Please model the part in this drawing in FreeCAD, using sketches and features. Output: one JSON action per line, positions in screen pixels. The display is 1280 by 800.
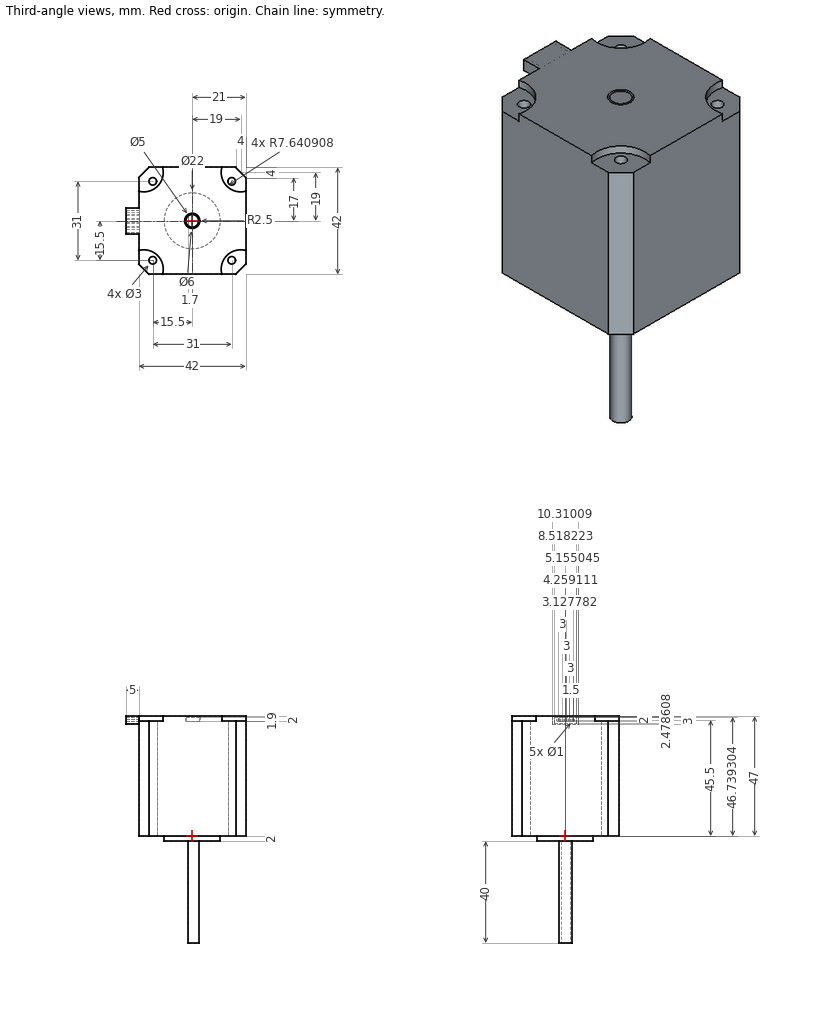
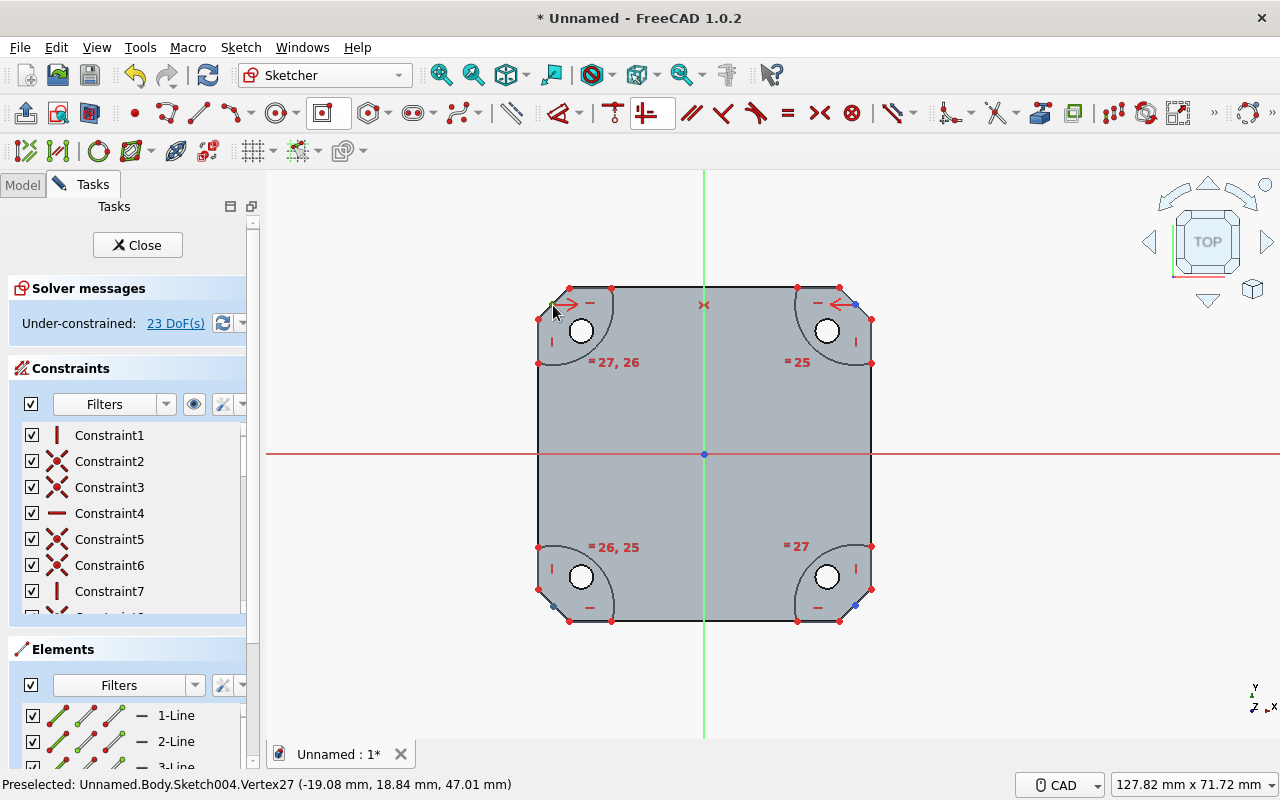
{"action": "left_click", "coordinate": [353, 454]}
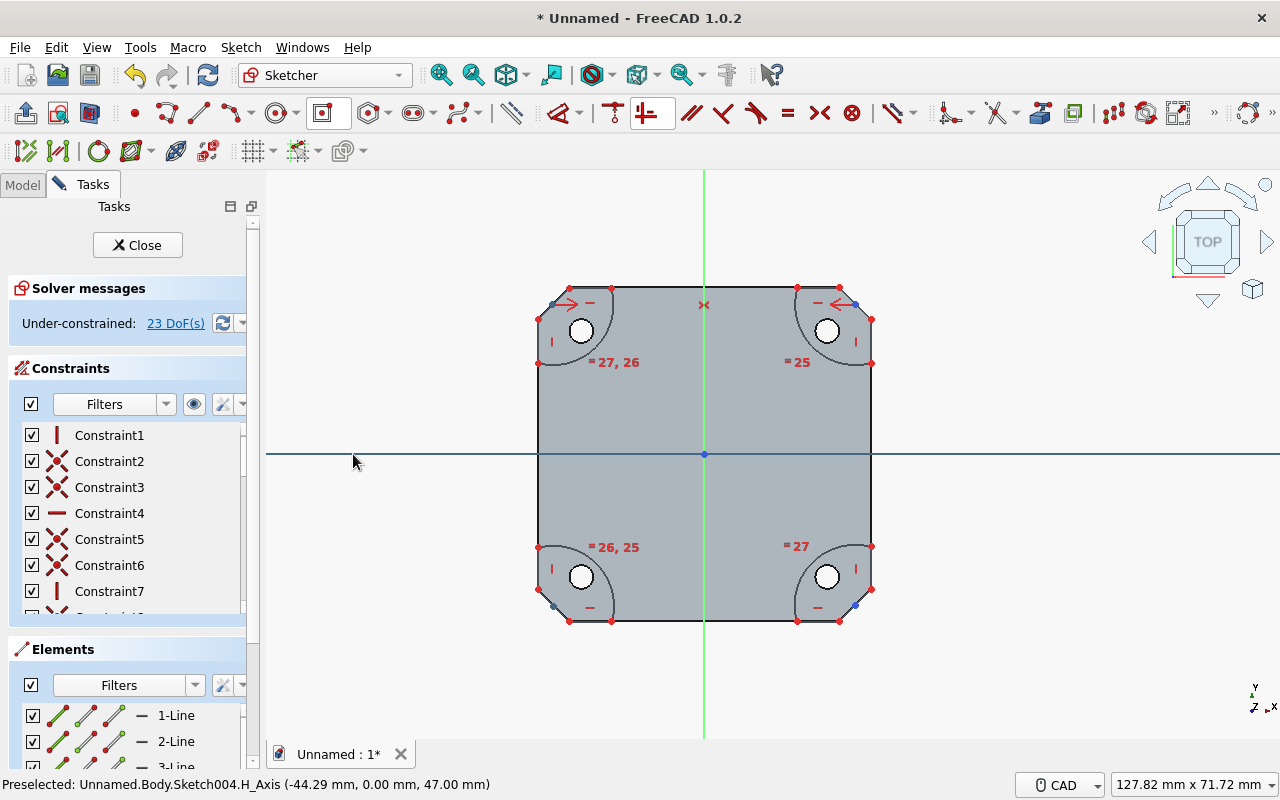
{"action": "left_click", "coordinate": [820, 114]}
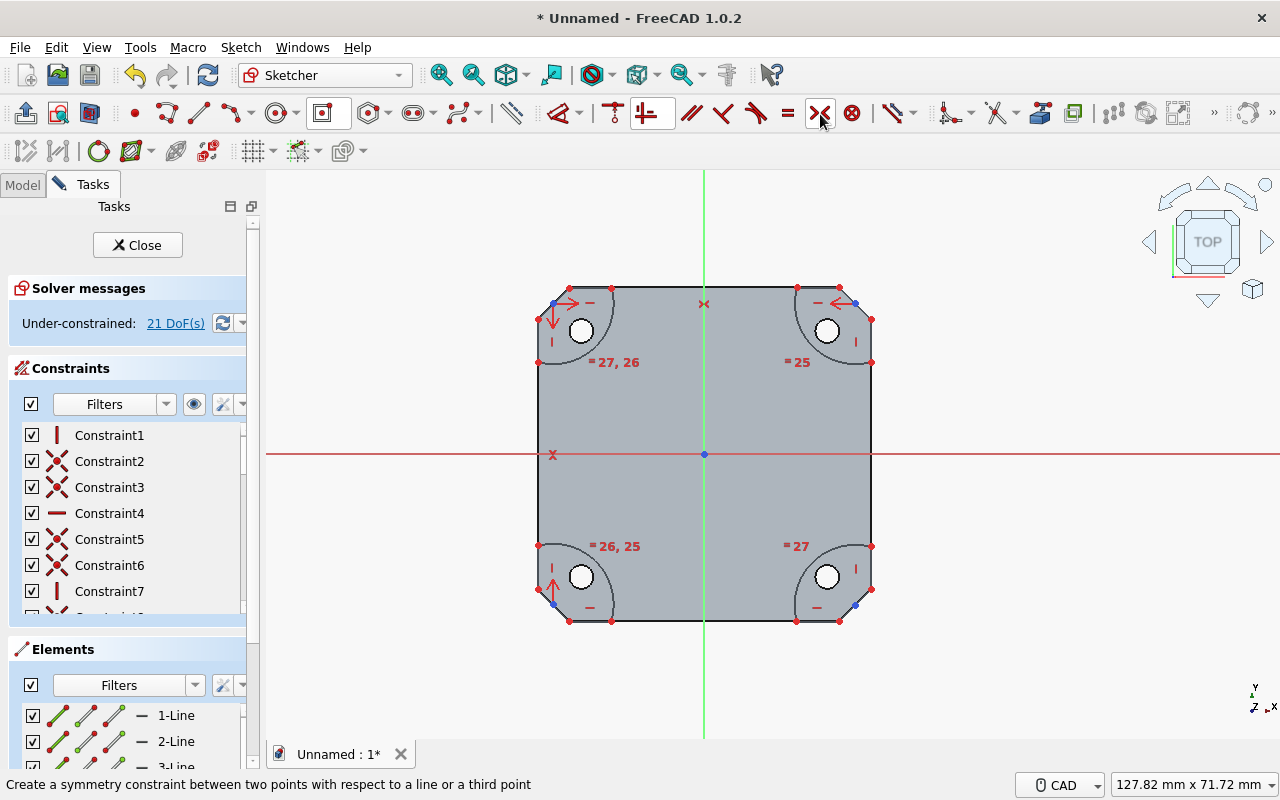
{"action": "left_click", "coordinate": [856, 304]}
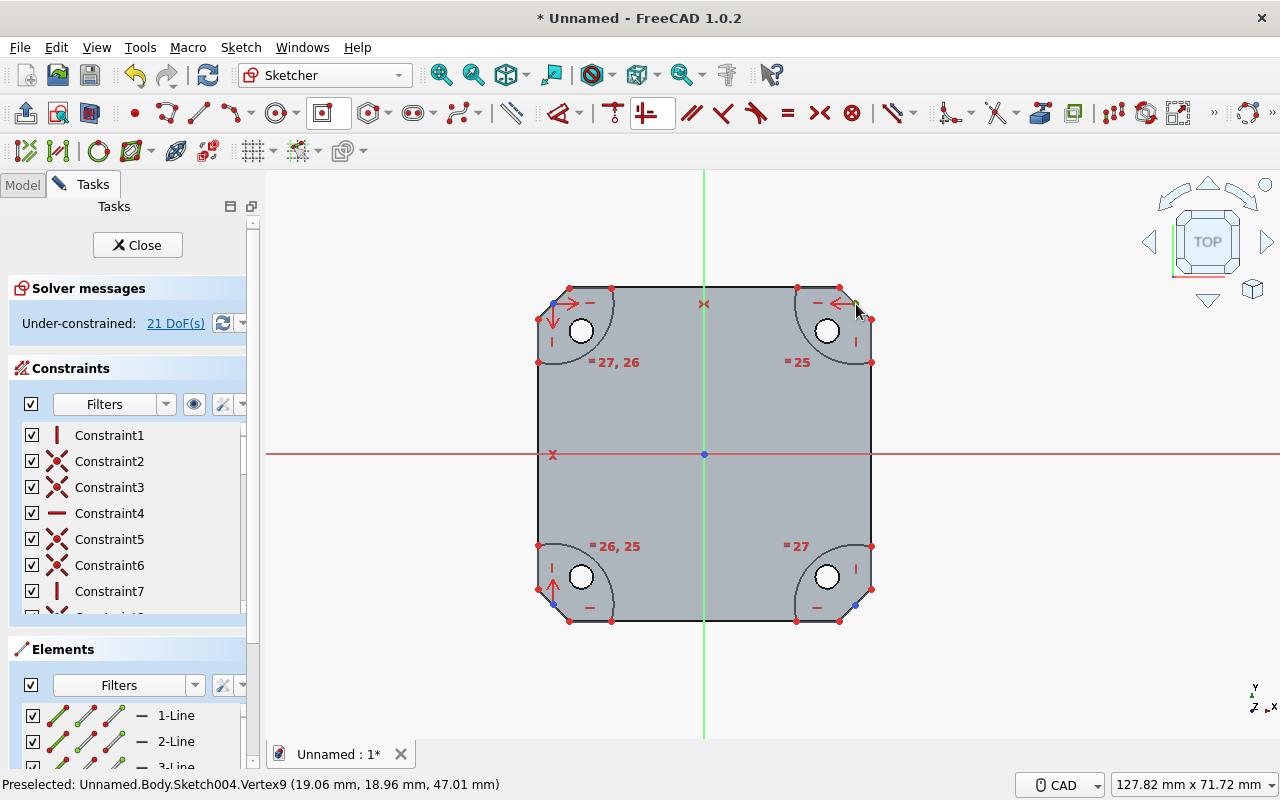
{"action": "left_click", "coordinate": [855, 605]}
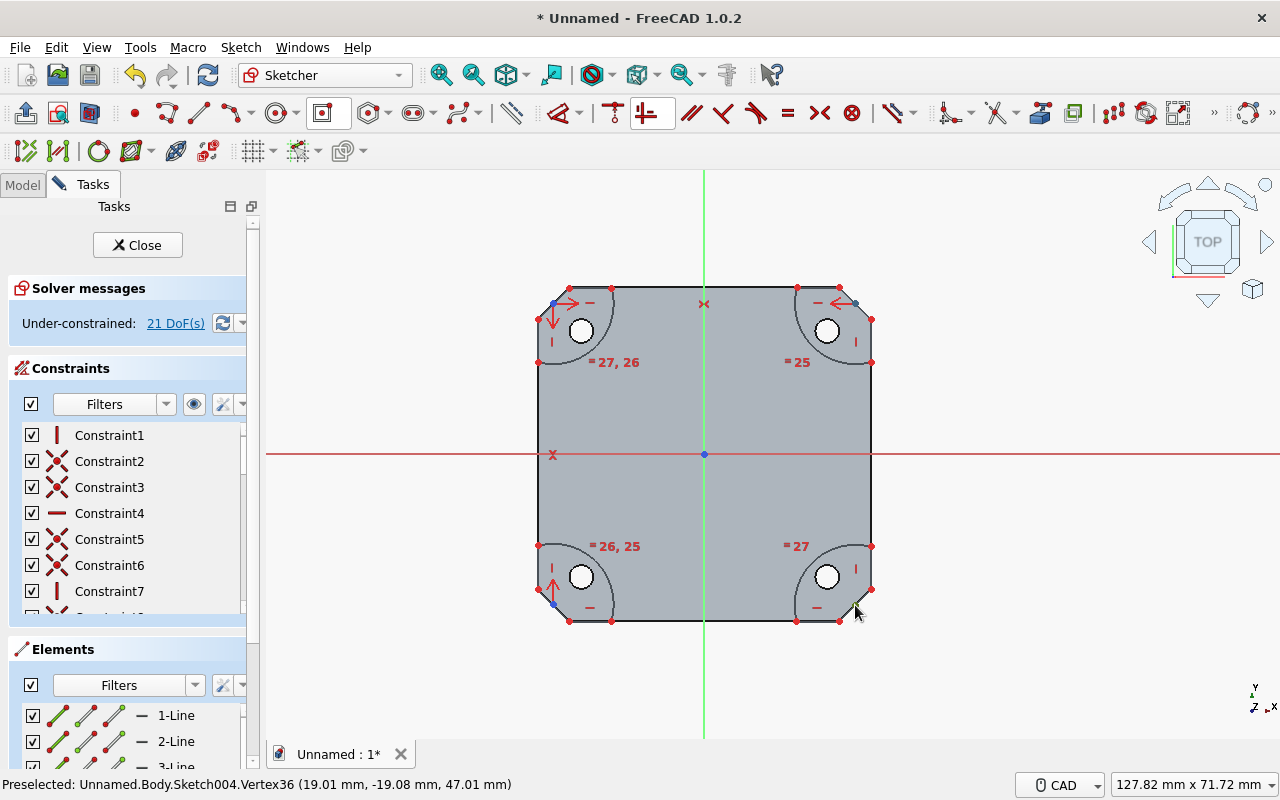
{"action": "left_click", "coordinate": [353, 454]}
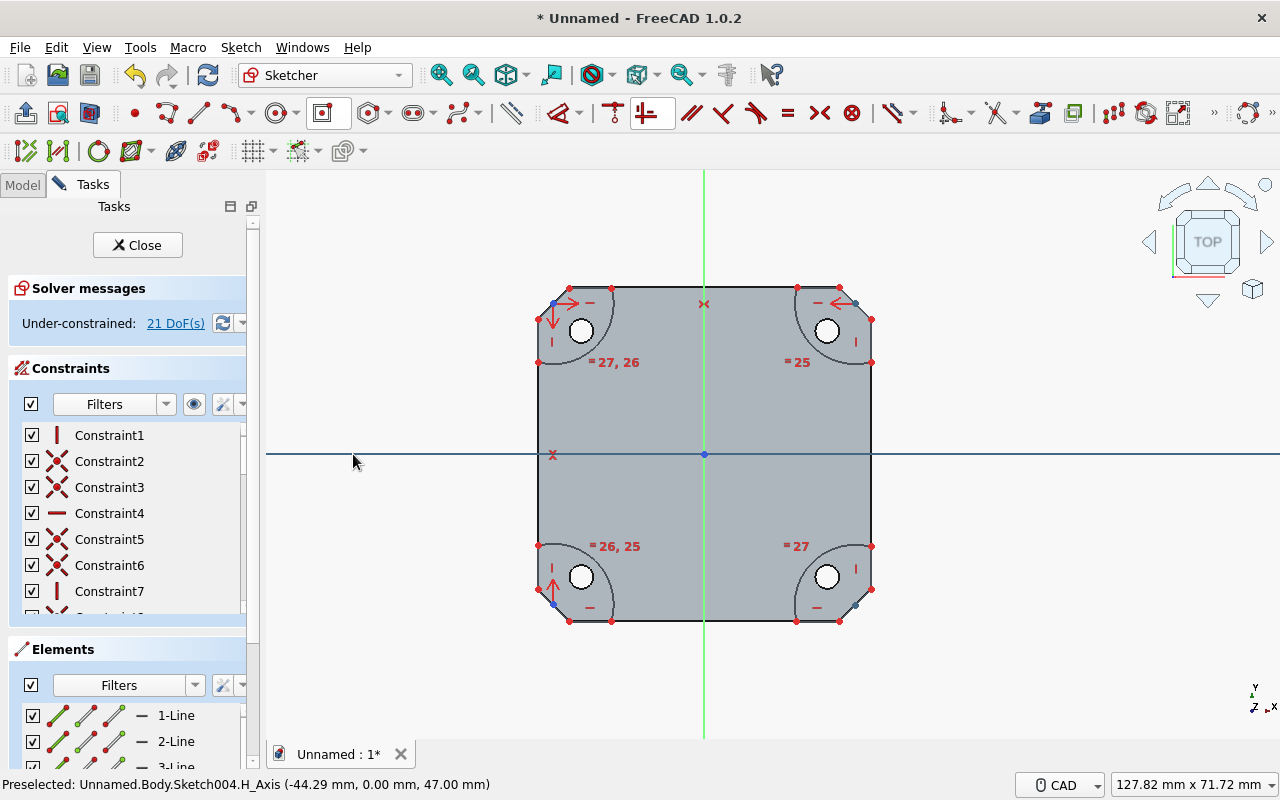
{"action": "left_click", "coordinate": [820, 114]}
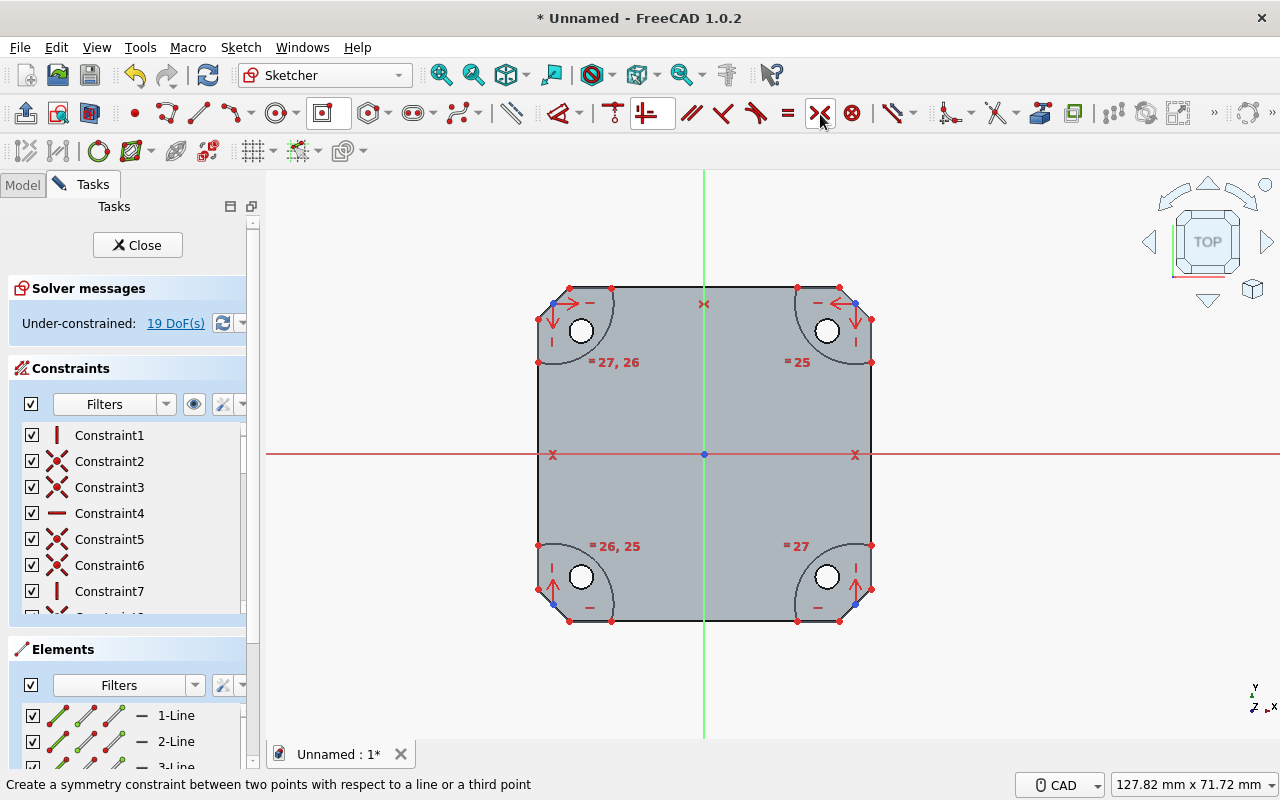
{"action": "left_click", "coordinate": [839, 288]}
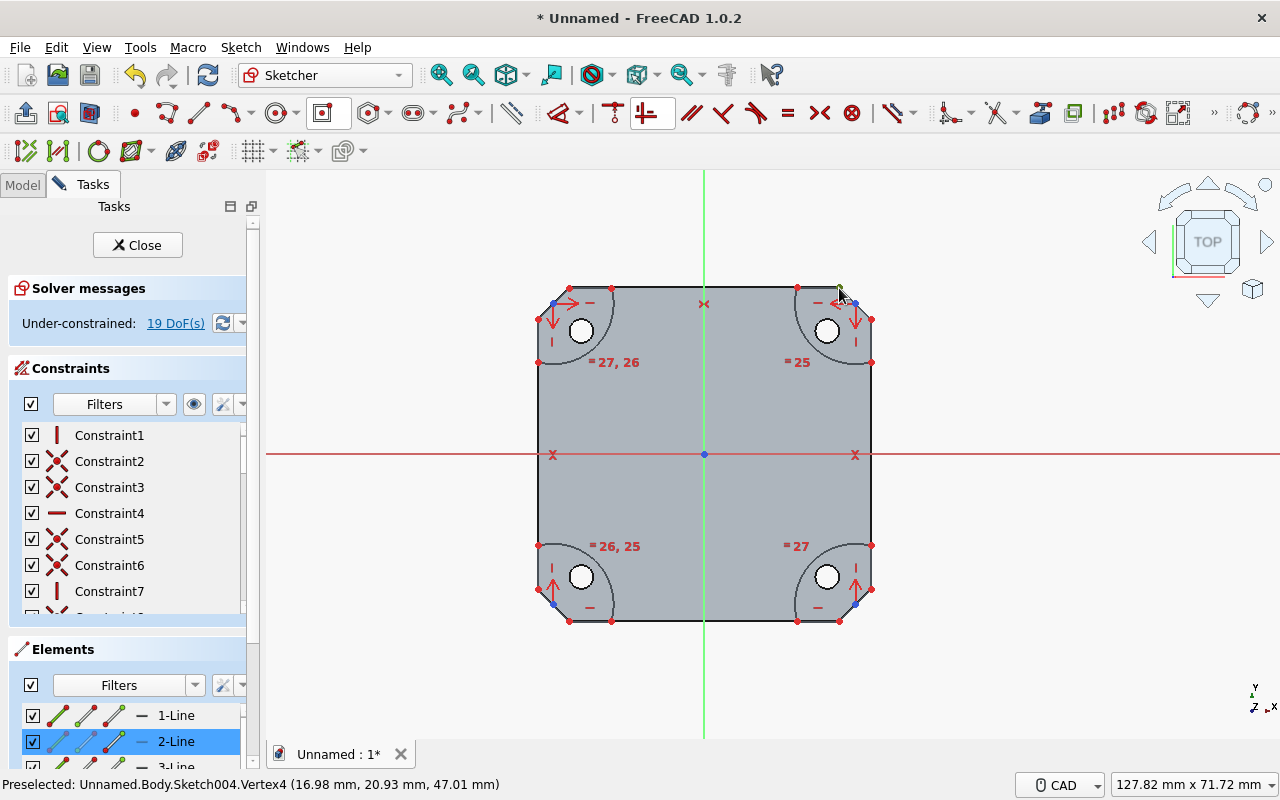
{"action": "left_click", "coordinate": [569, 288]}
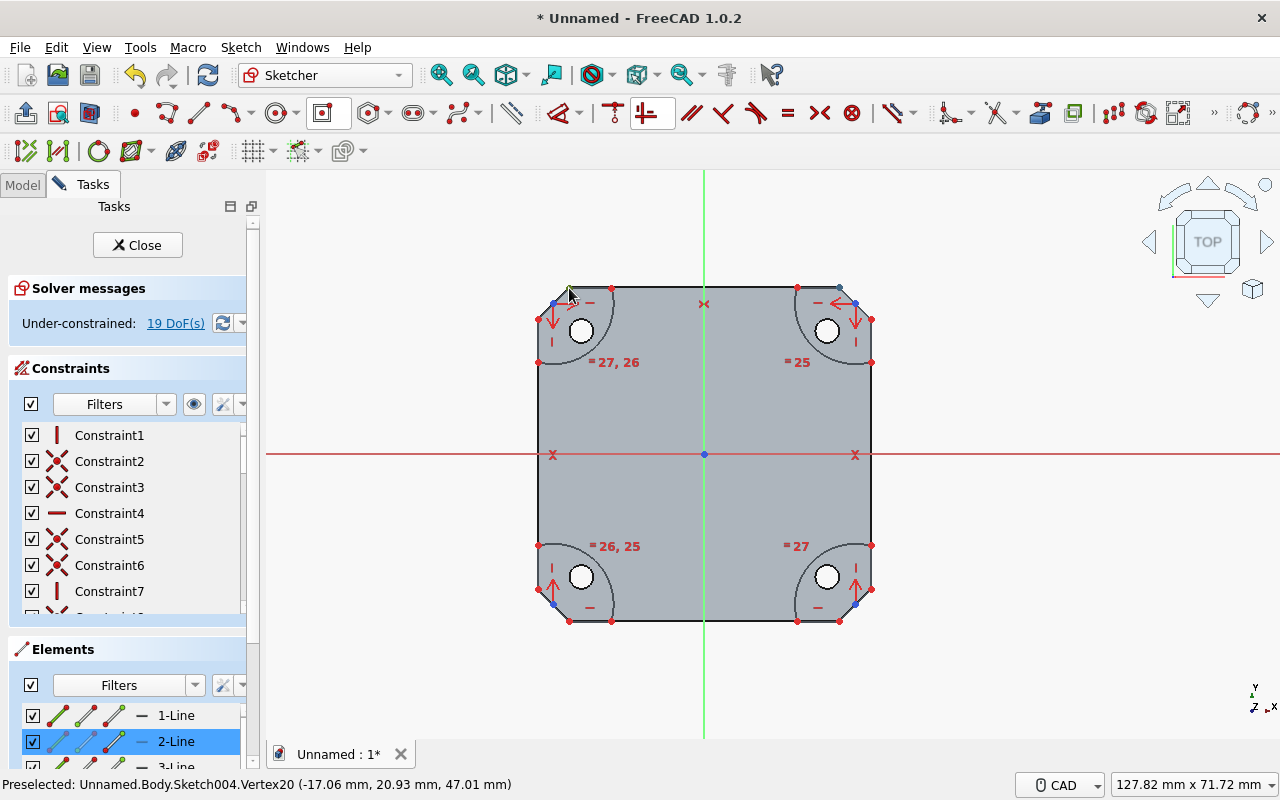
{"action": "left_click", "coordinate": [704, 674]}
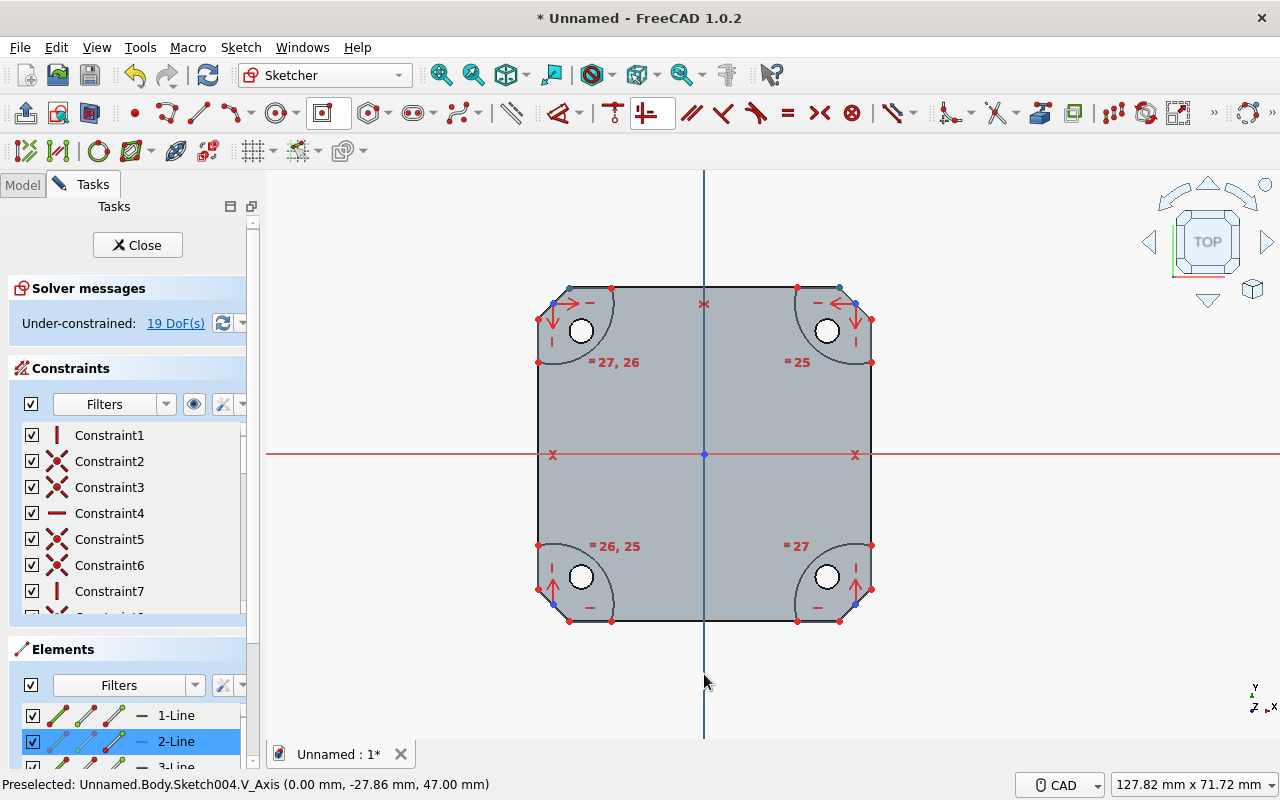
{"action": "left_click", "coordinate": [820, 114]}